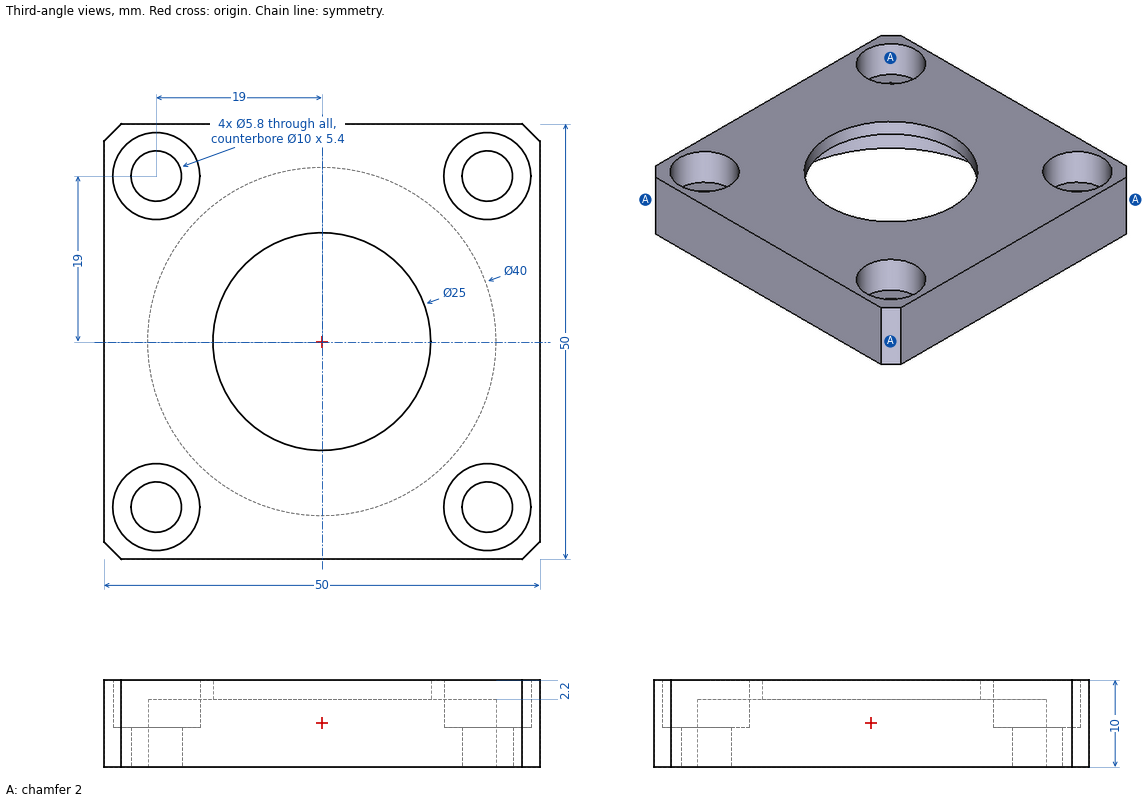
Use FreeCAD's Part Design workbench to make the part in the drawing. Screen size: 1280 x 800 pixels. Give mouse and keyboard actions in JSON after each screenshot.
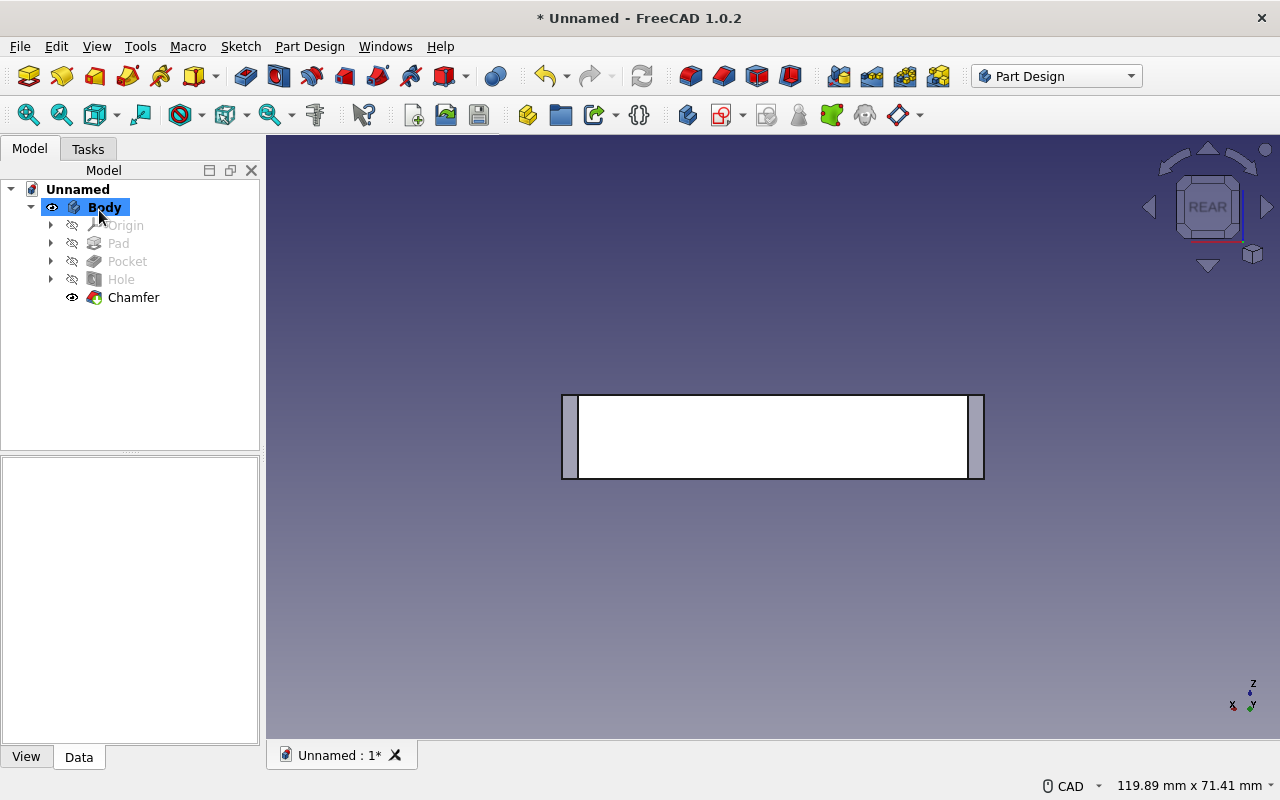
{"action": "left_click", "coordinate": [29, 116]}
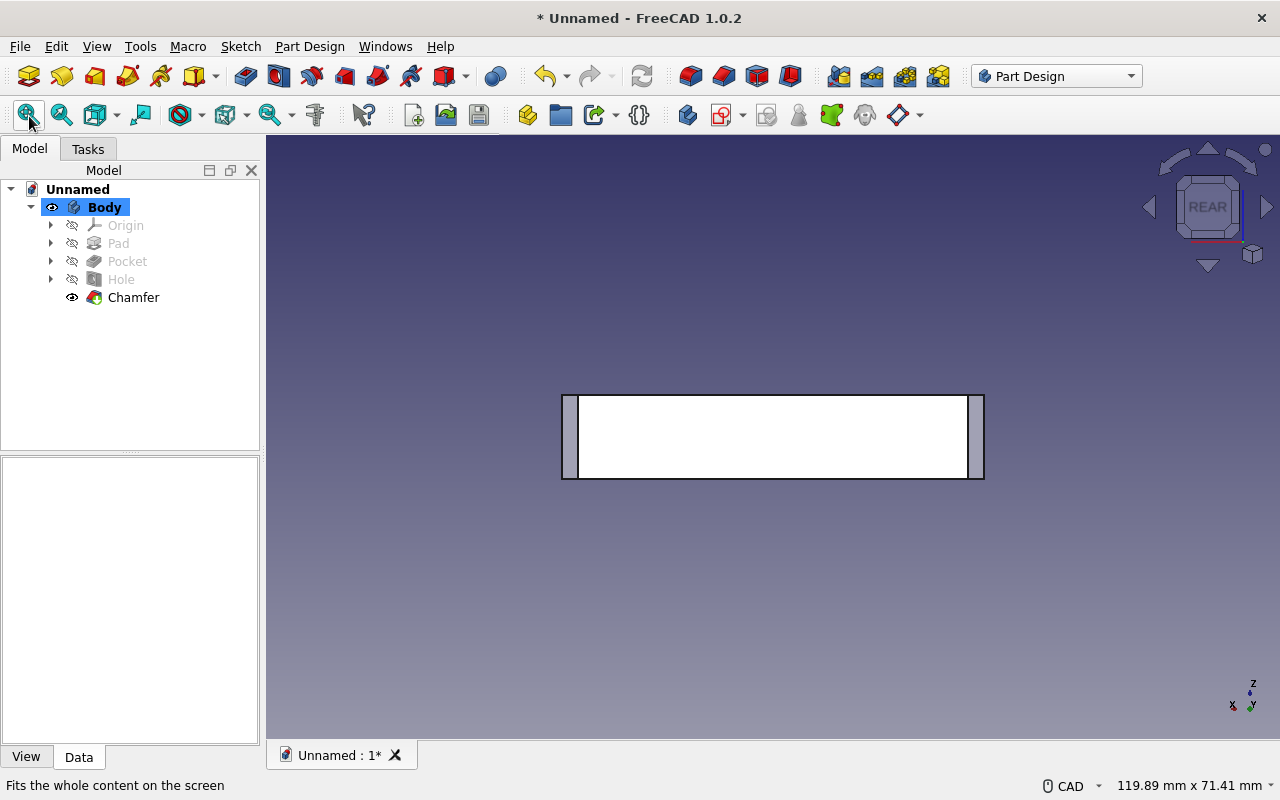
{"action": "key", "text": "0"}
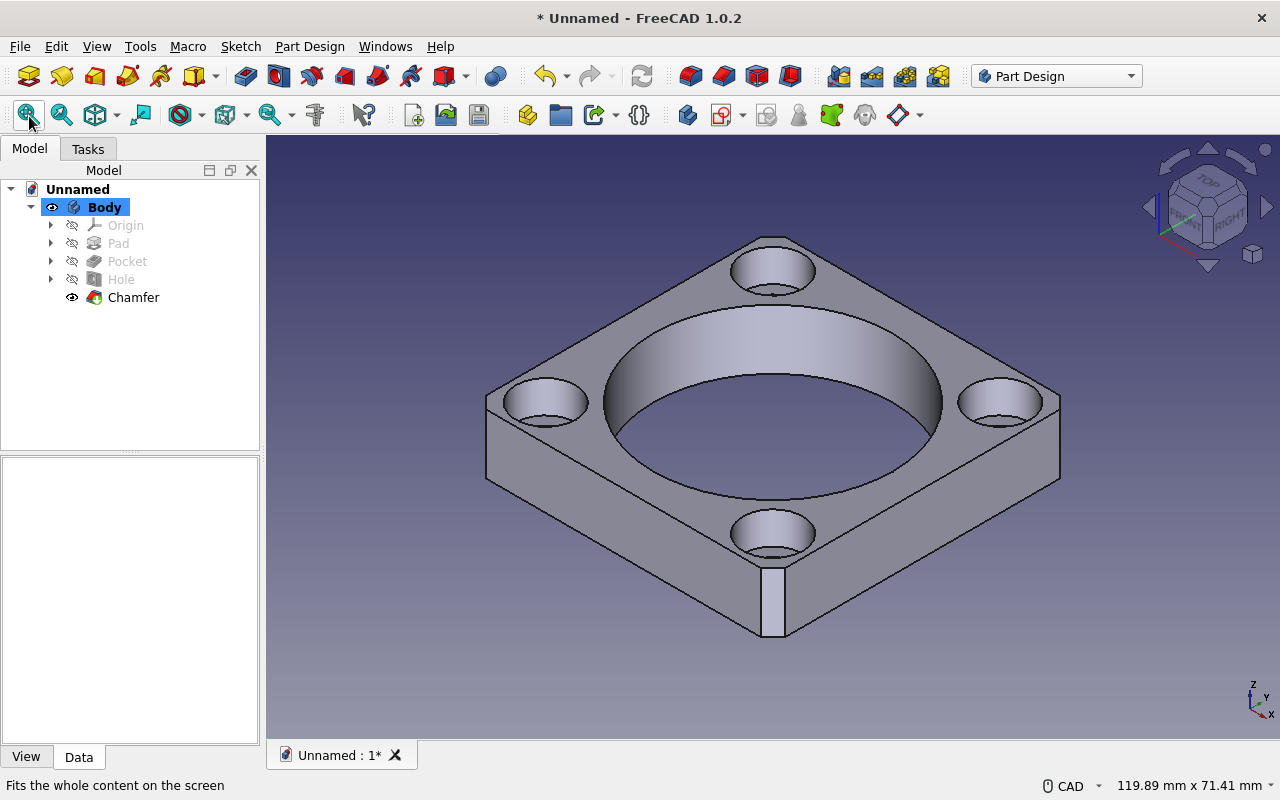
{"action": "left_click", "coordinate": [944, 451]}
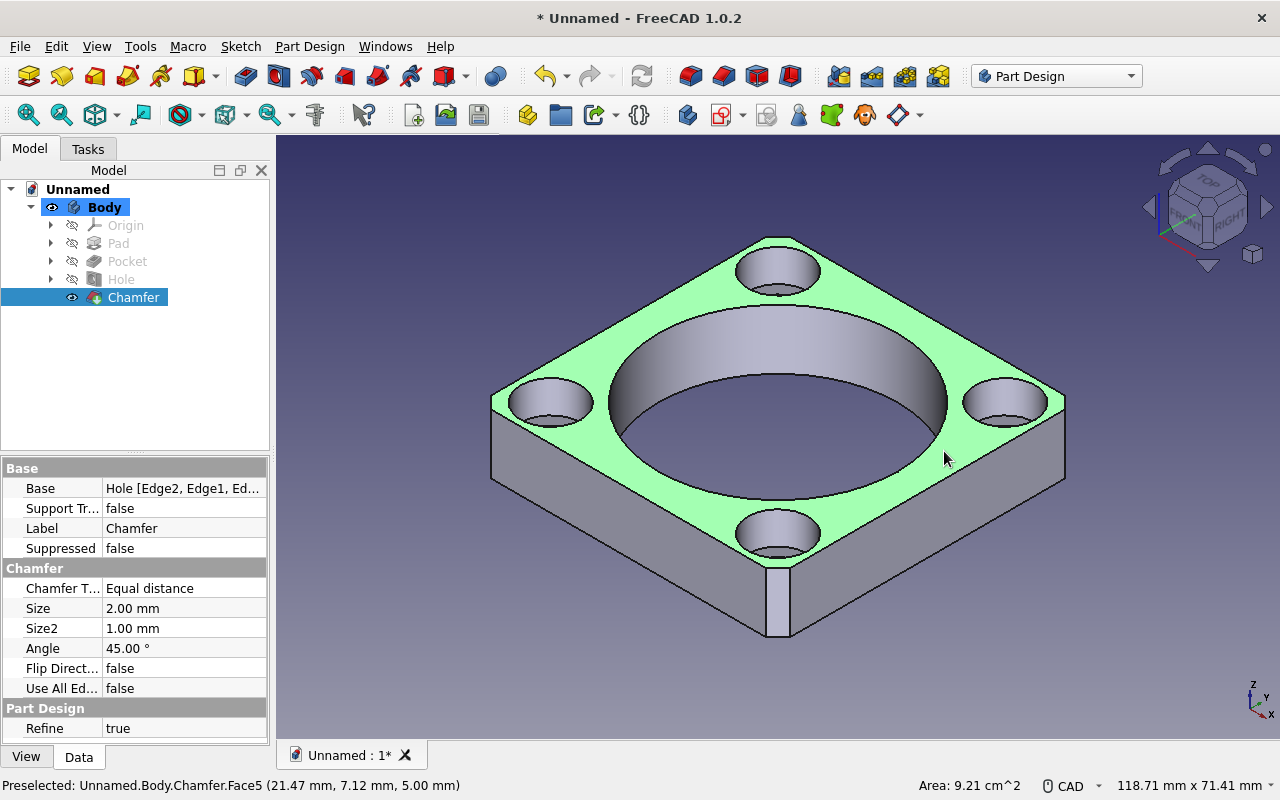
{"action": "left_click", "coordinate": [720, 116]}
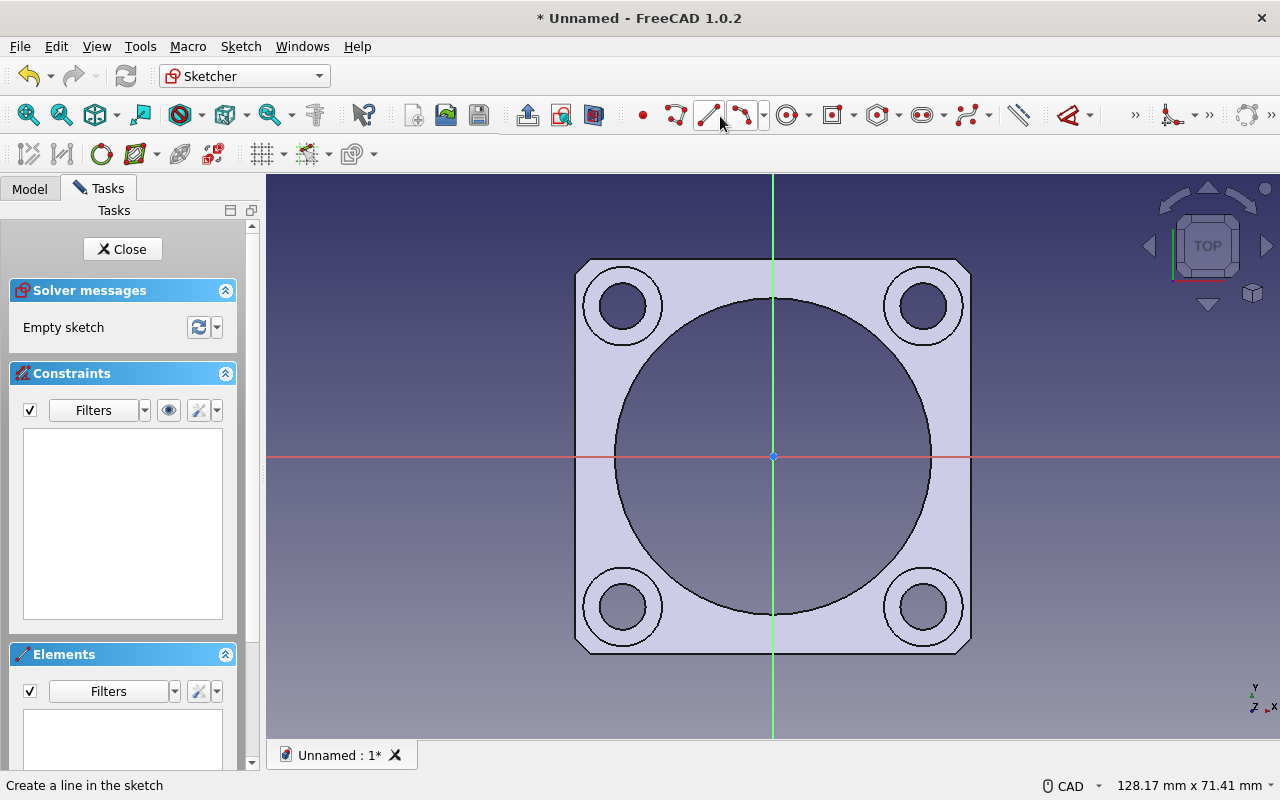
{"action": "left_click", "coordinate": [786, 116]}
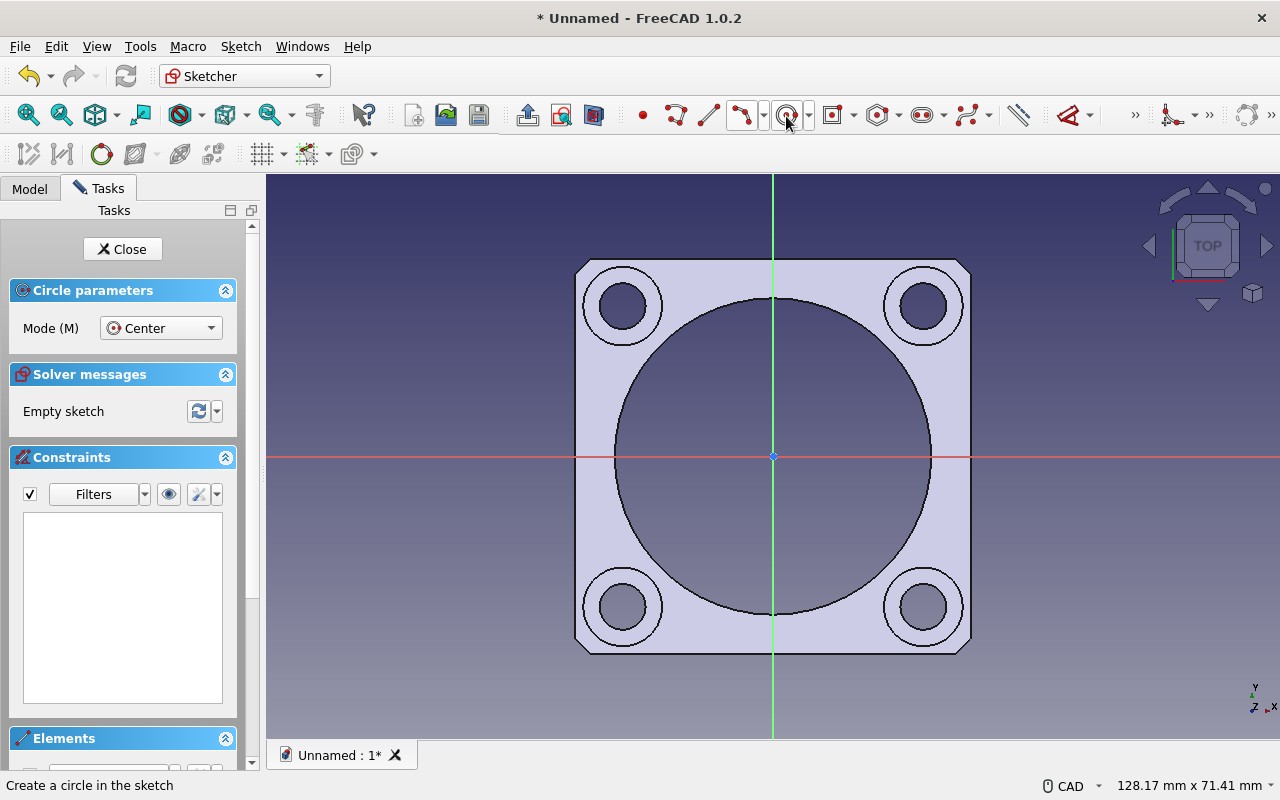
{"action": "left_click", "coordinate": [773, 457]}
{"action": "mouse_move", "coordinate": [885, 345]}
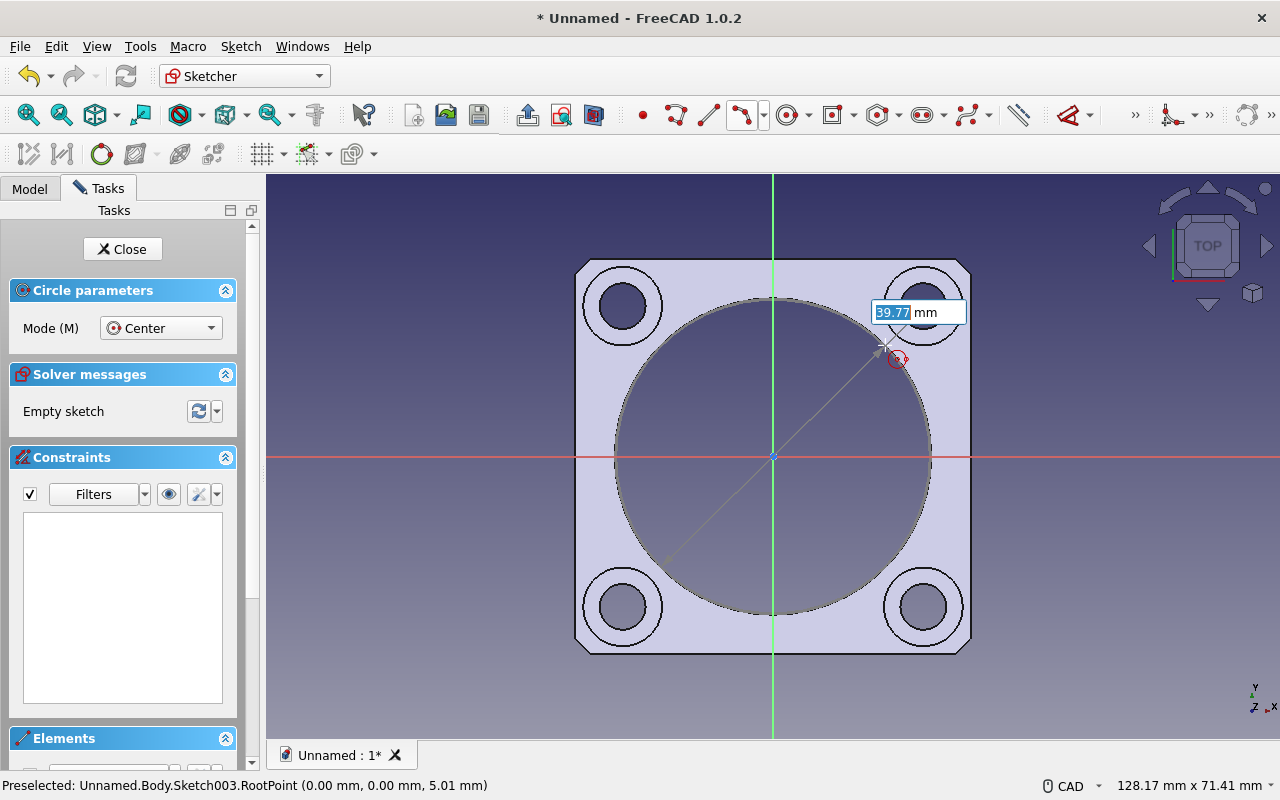
{"action": "type", "text": "40"}
{"action": "key", "text": "Return"}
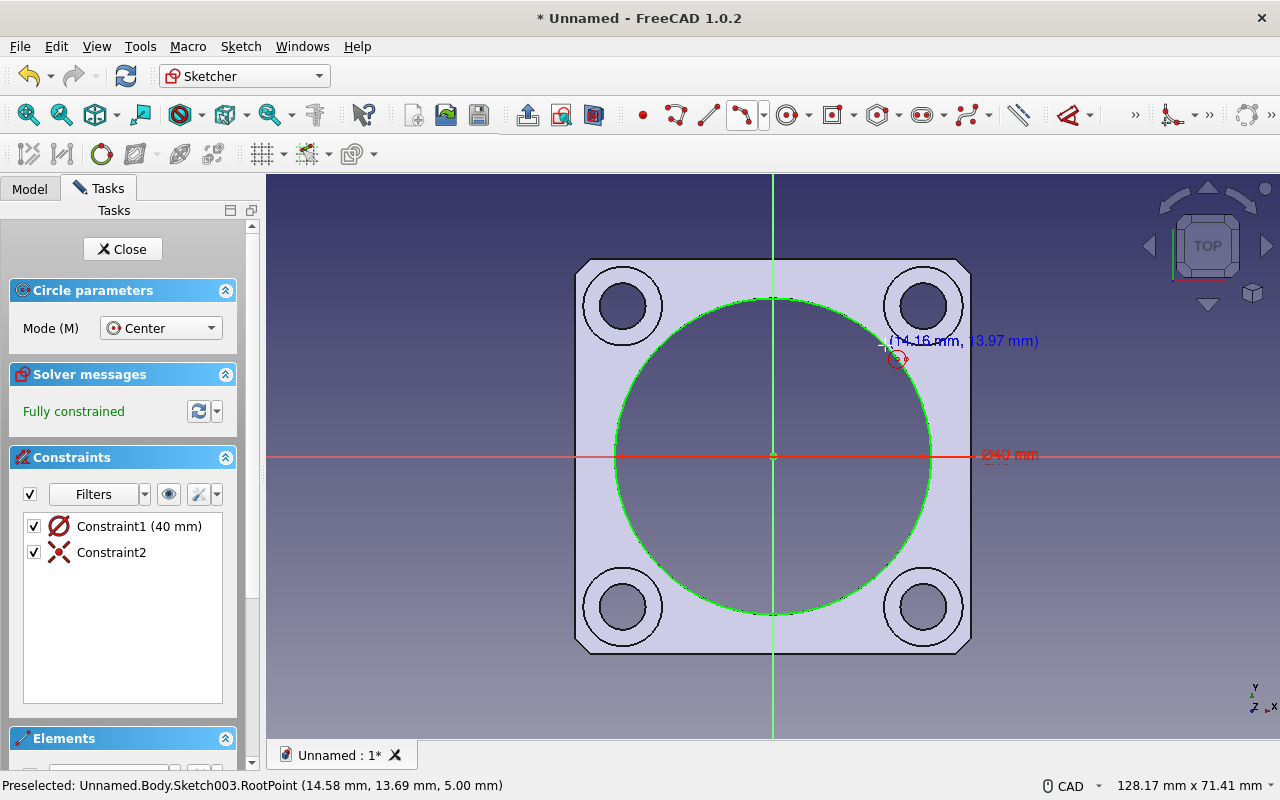
{"action": "left_click", "coordinate": [773, 457]}
{"action": "mouse_move", "coordinate": [843, 387]}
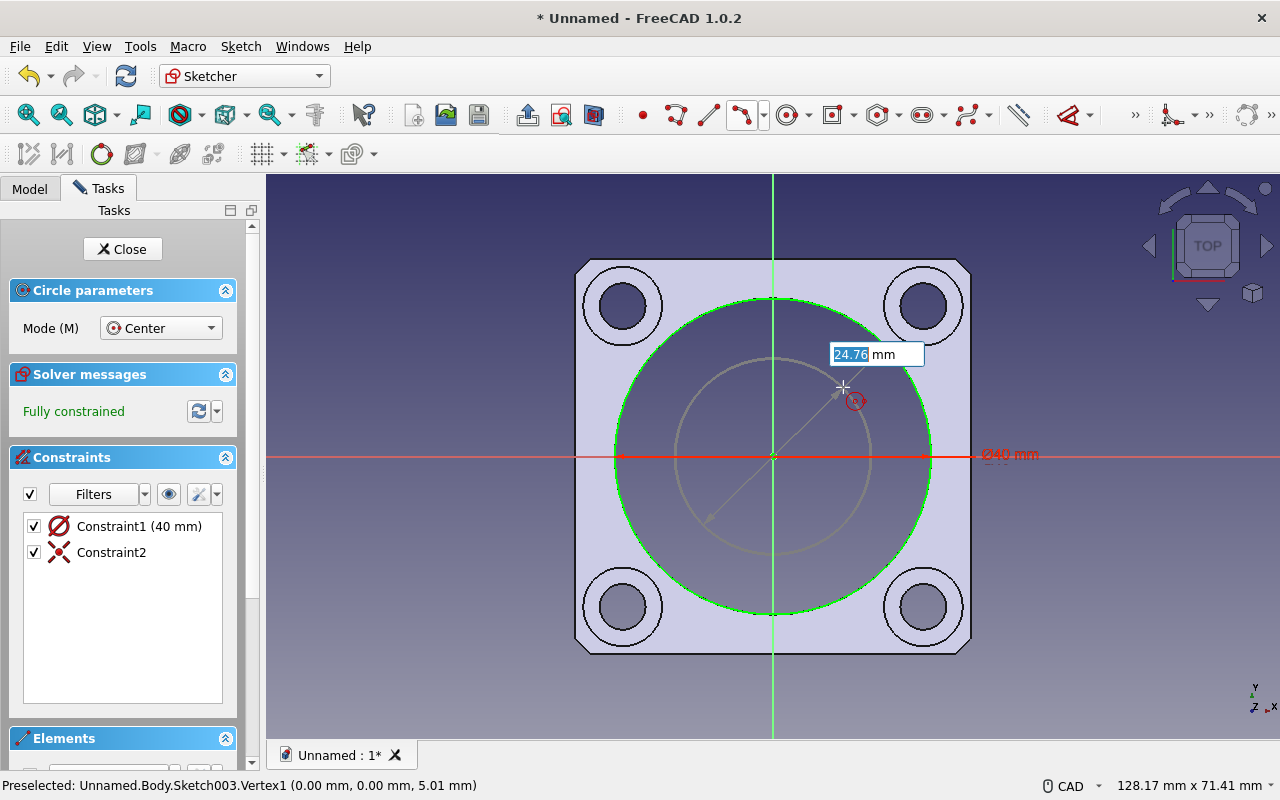
{"action": "type", "text": "25"}
{"action": "key", "text": "Return"}
{"action": "key", "text": "Escape"}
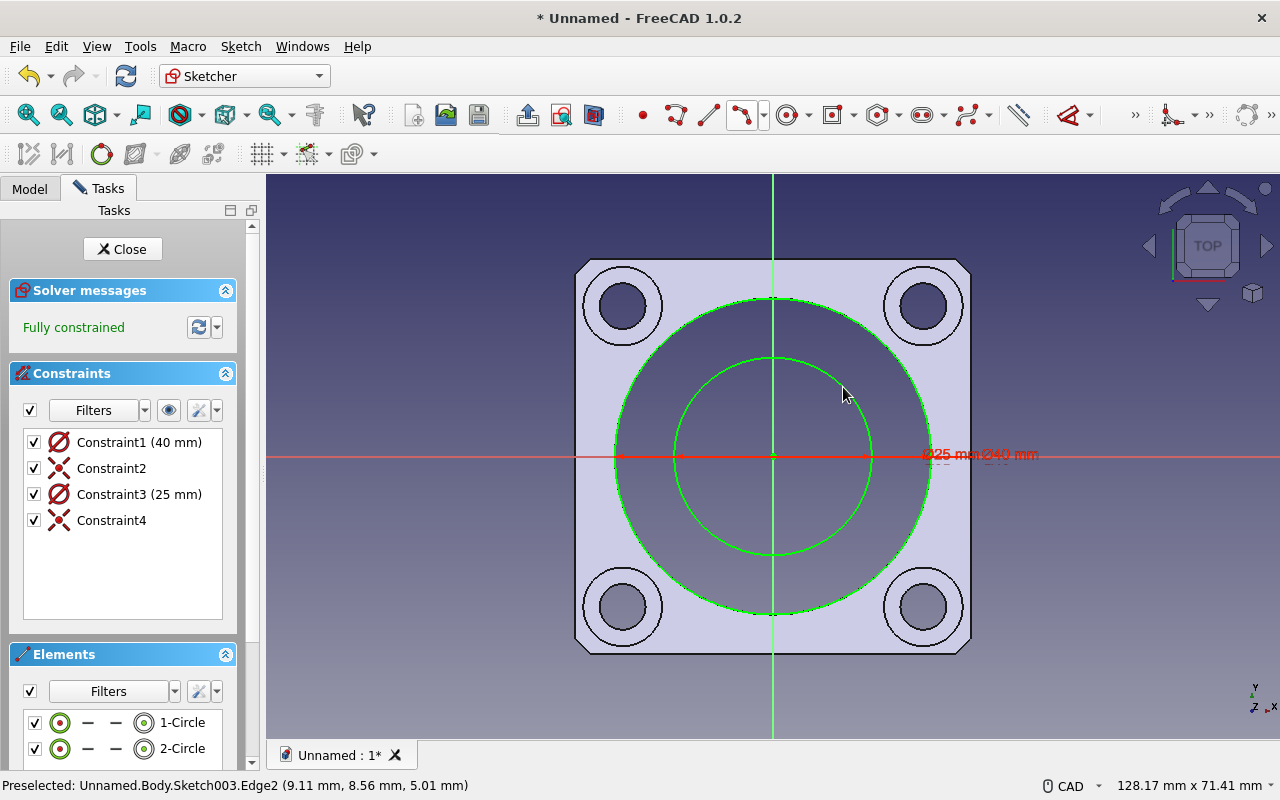
{"action": "left_click", "coordinate": [123, 249]}